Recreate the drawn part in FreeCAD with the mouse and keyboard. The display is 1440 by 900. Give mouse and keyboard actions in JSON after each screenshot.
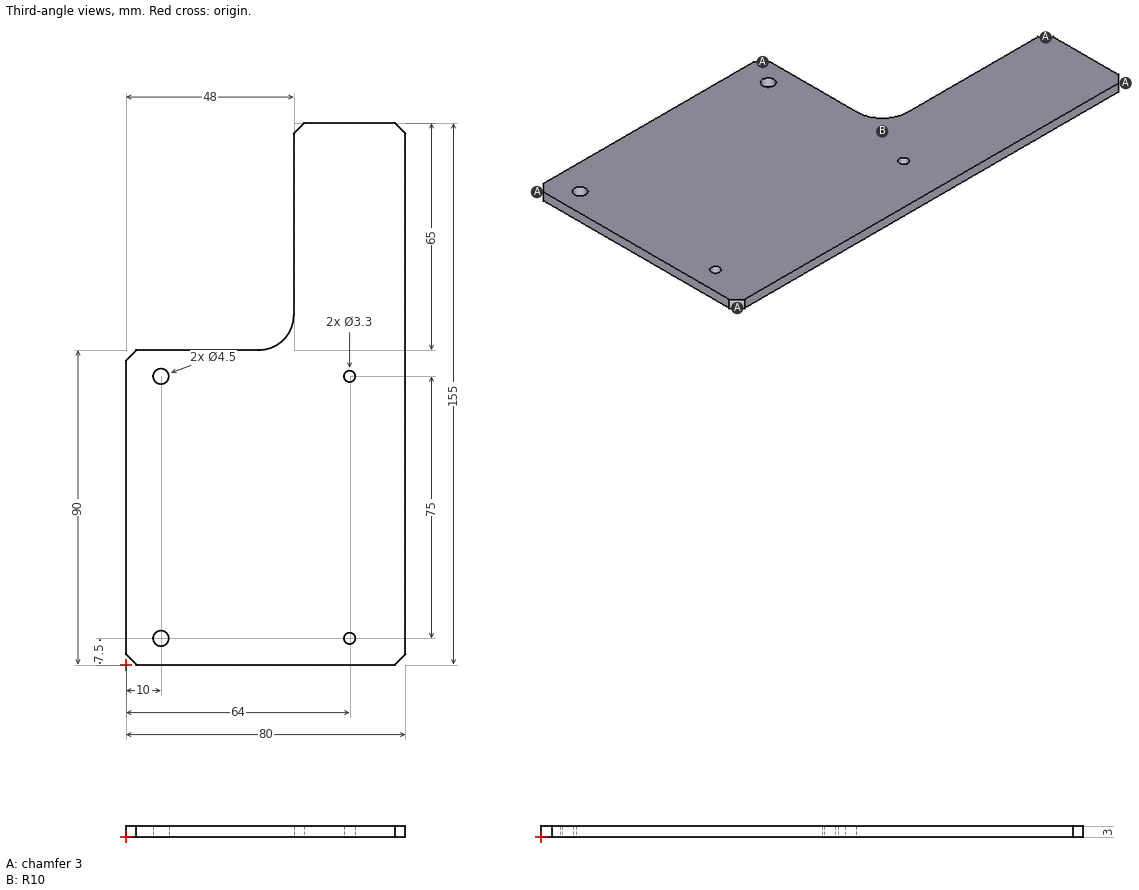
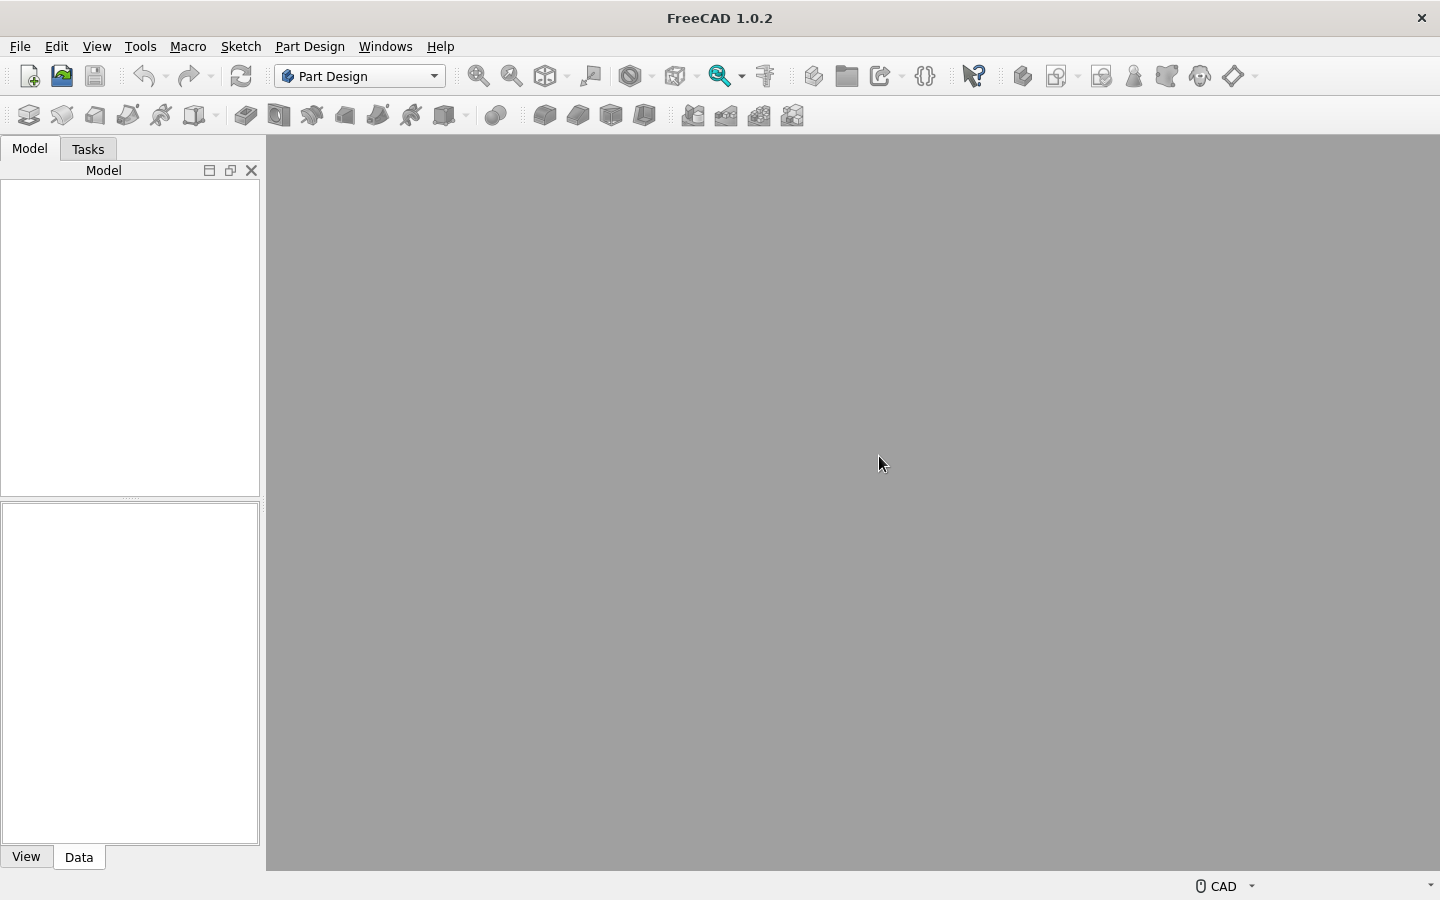
{"action": "left_click", "coordinate": [29, 76]}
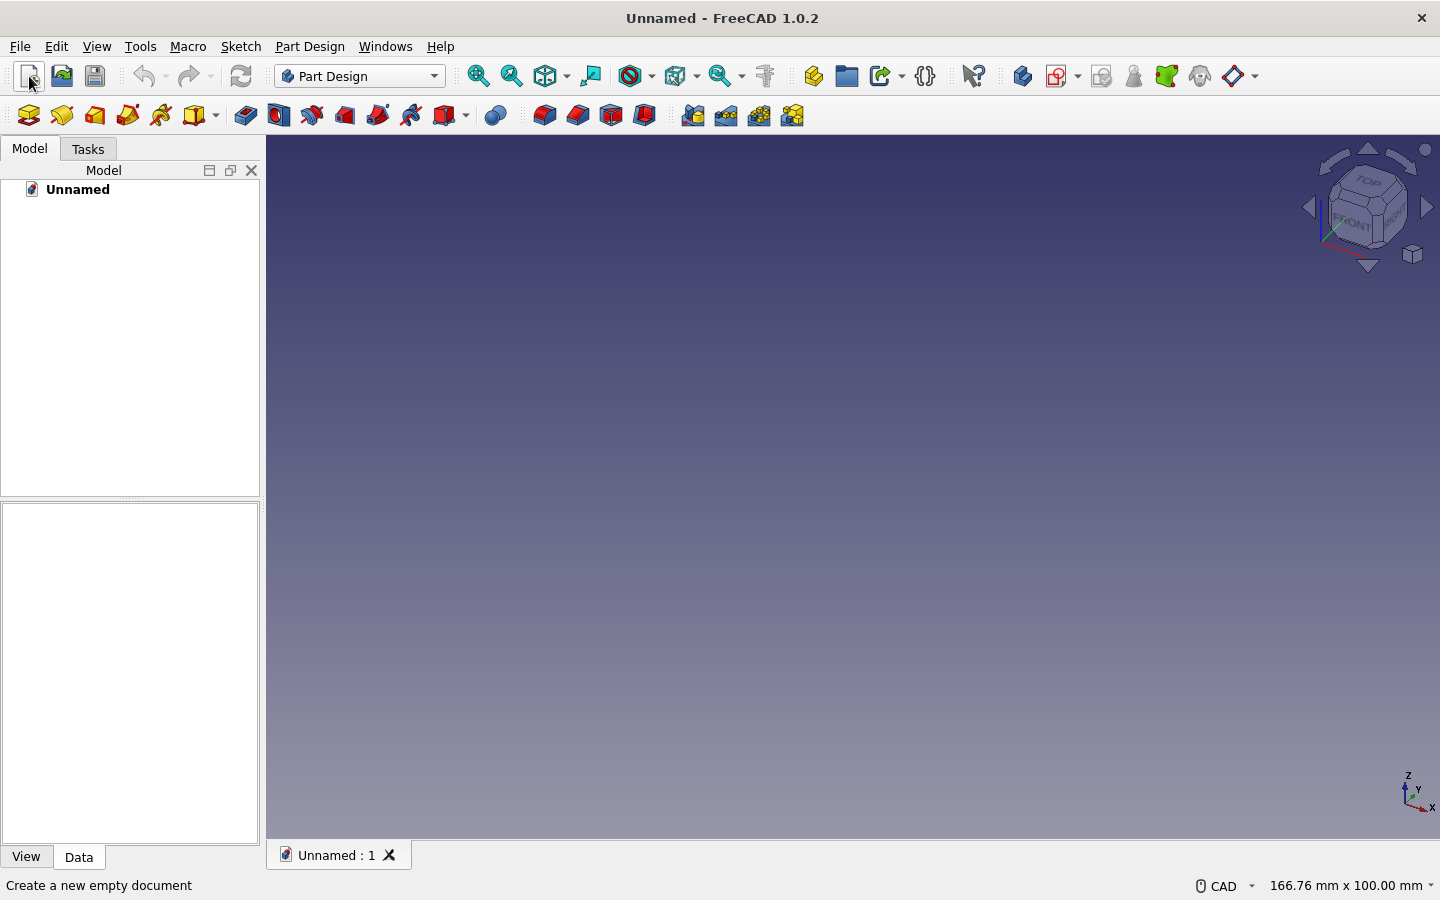
{"action": "left_click", "coordinate": [1056, 76]}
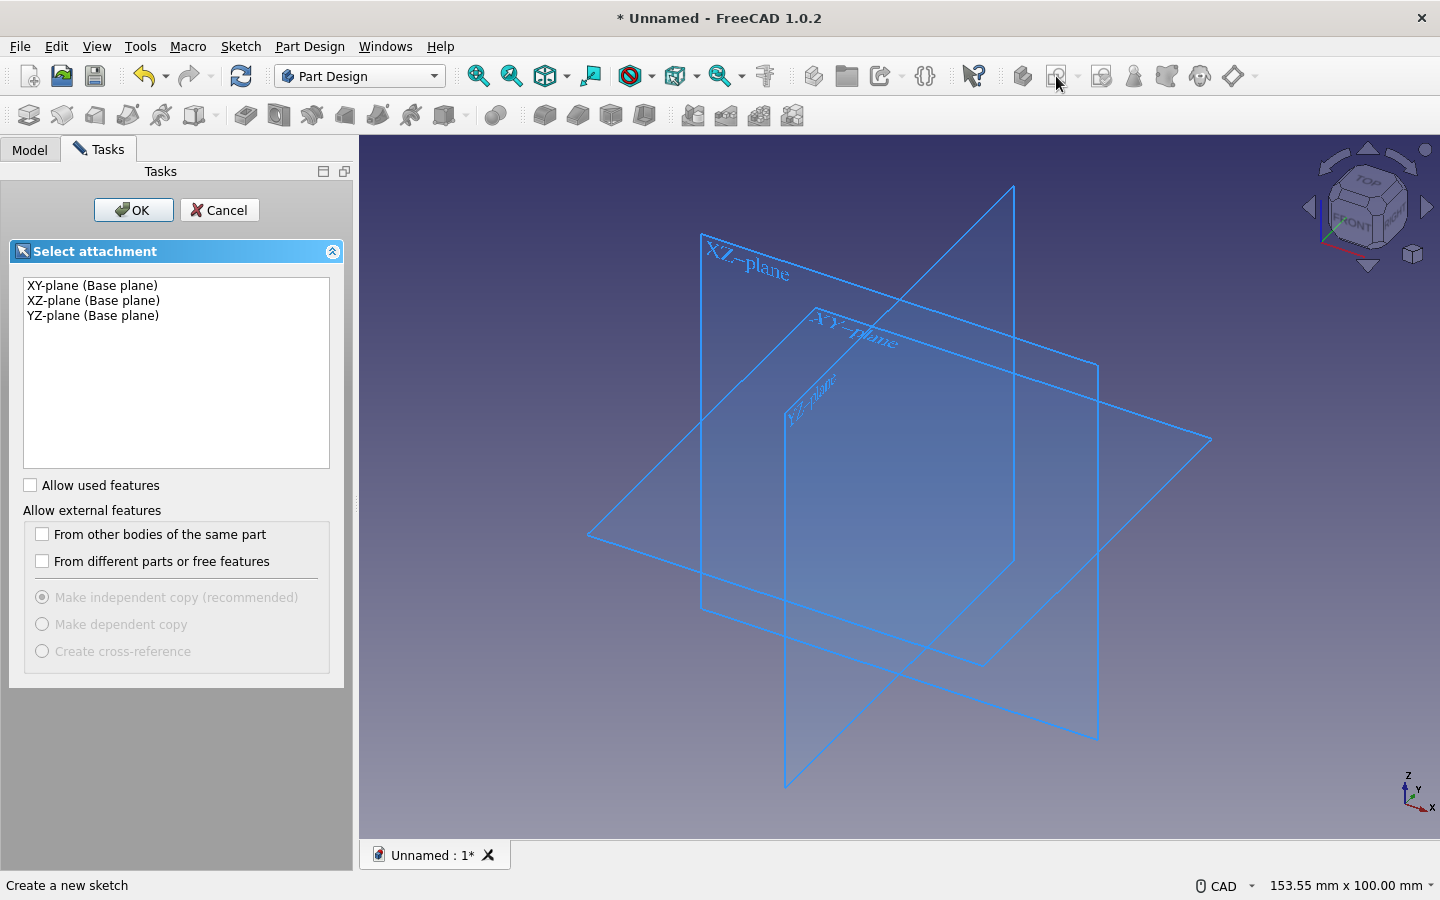
{"action": "left_click", "coordinate": [84, 286]}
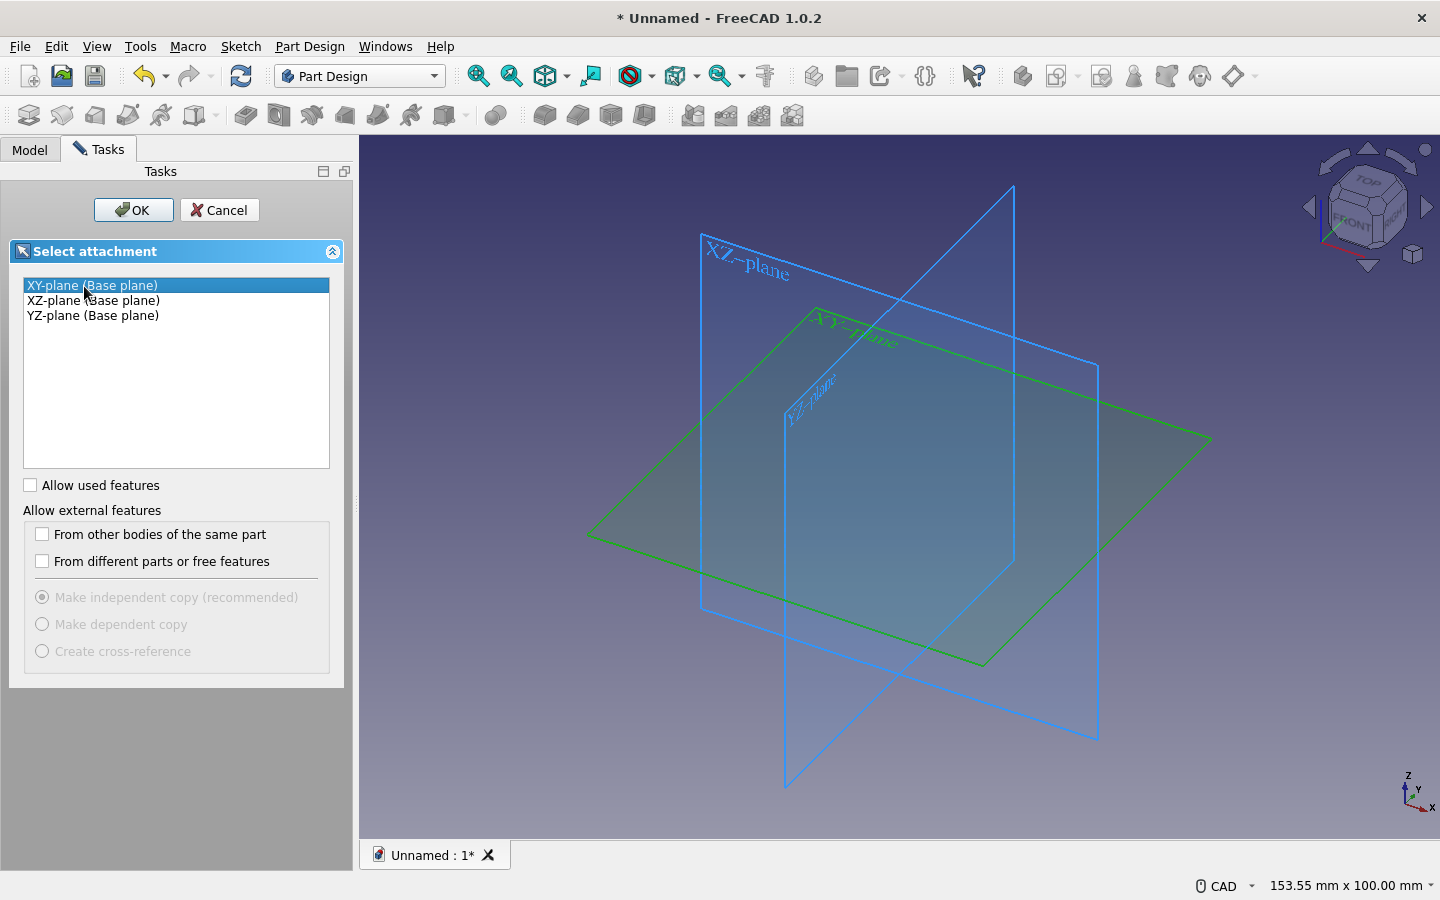
{"action": "left_click", "coordinate": [134, 210]}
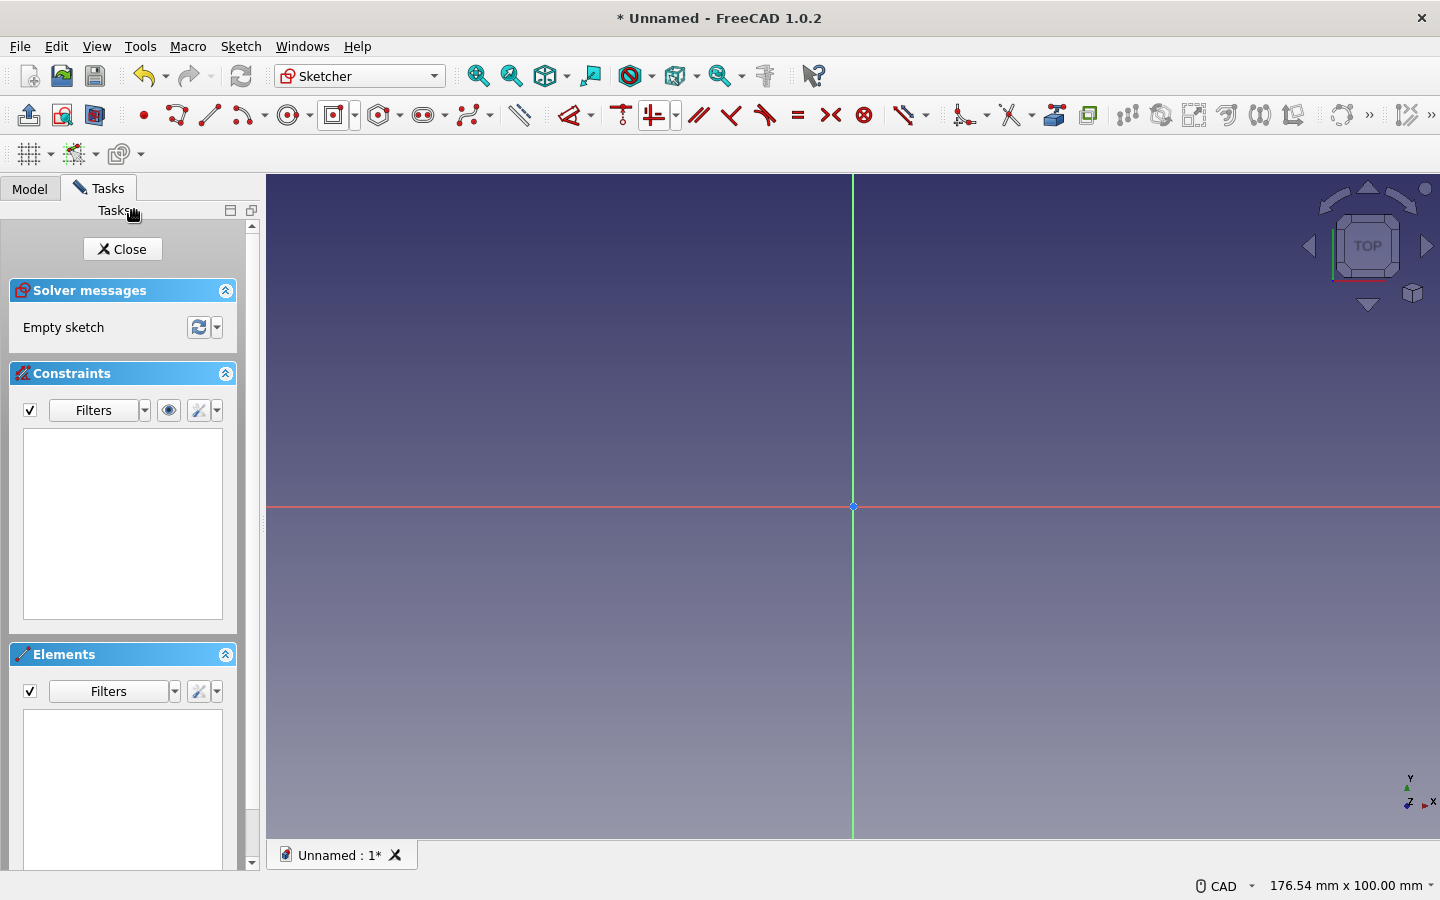
{"action": "scroll", "coordinate": [590, 806], "scroll_direction": "down", "scroll_amount": 5}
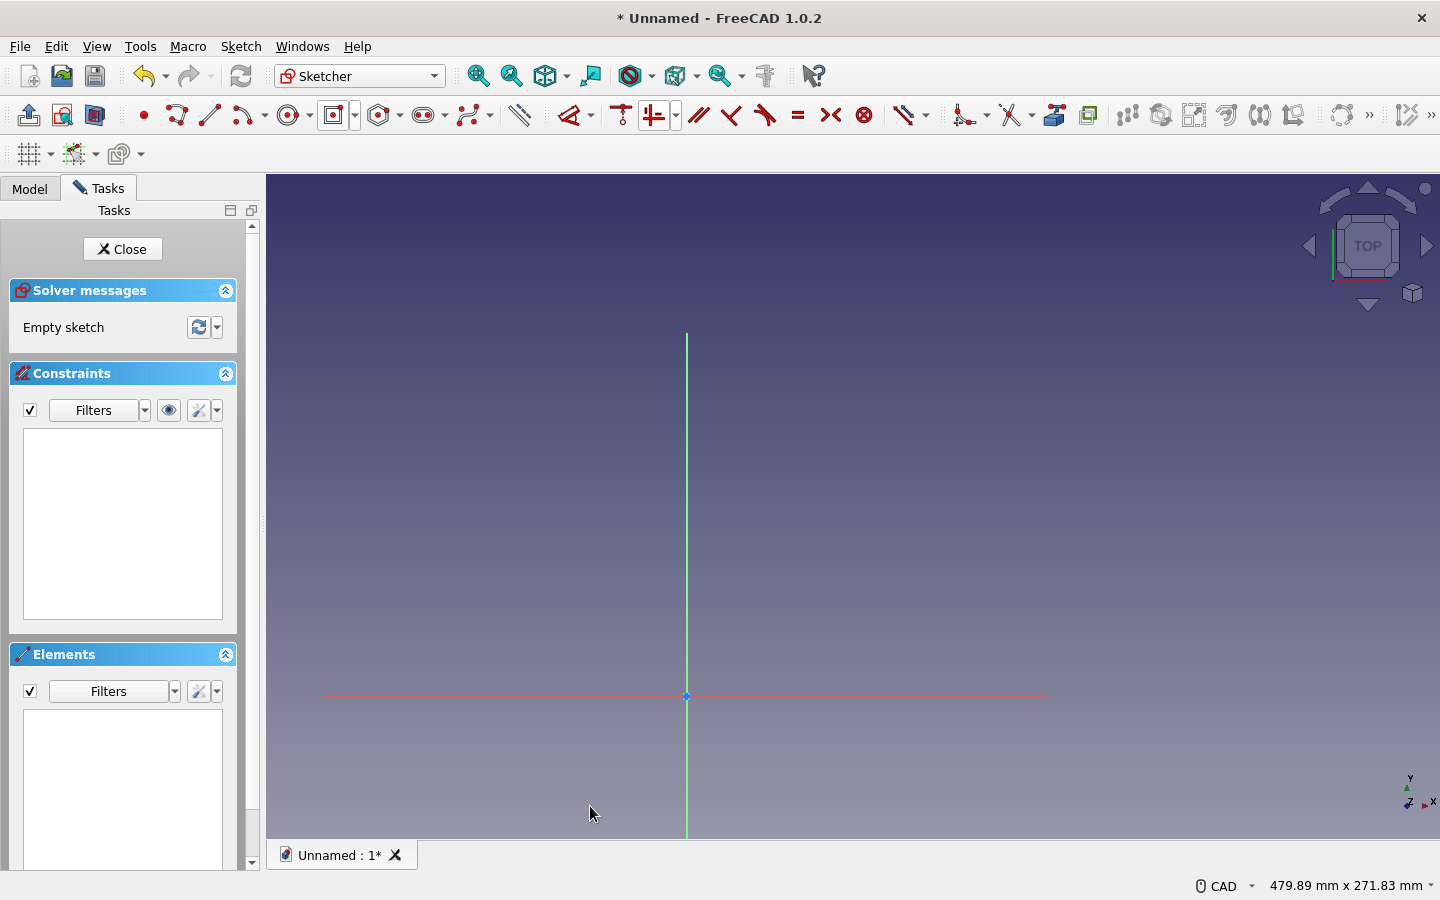
{"action": "left_click", "coordinate": [354, 116]}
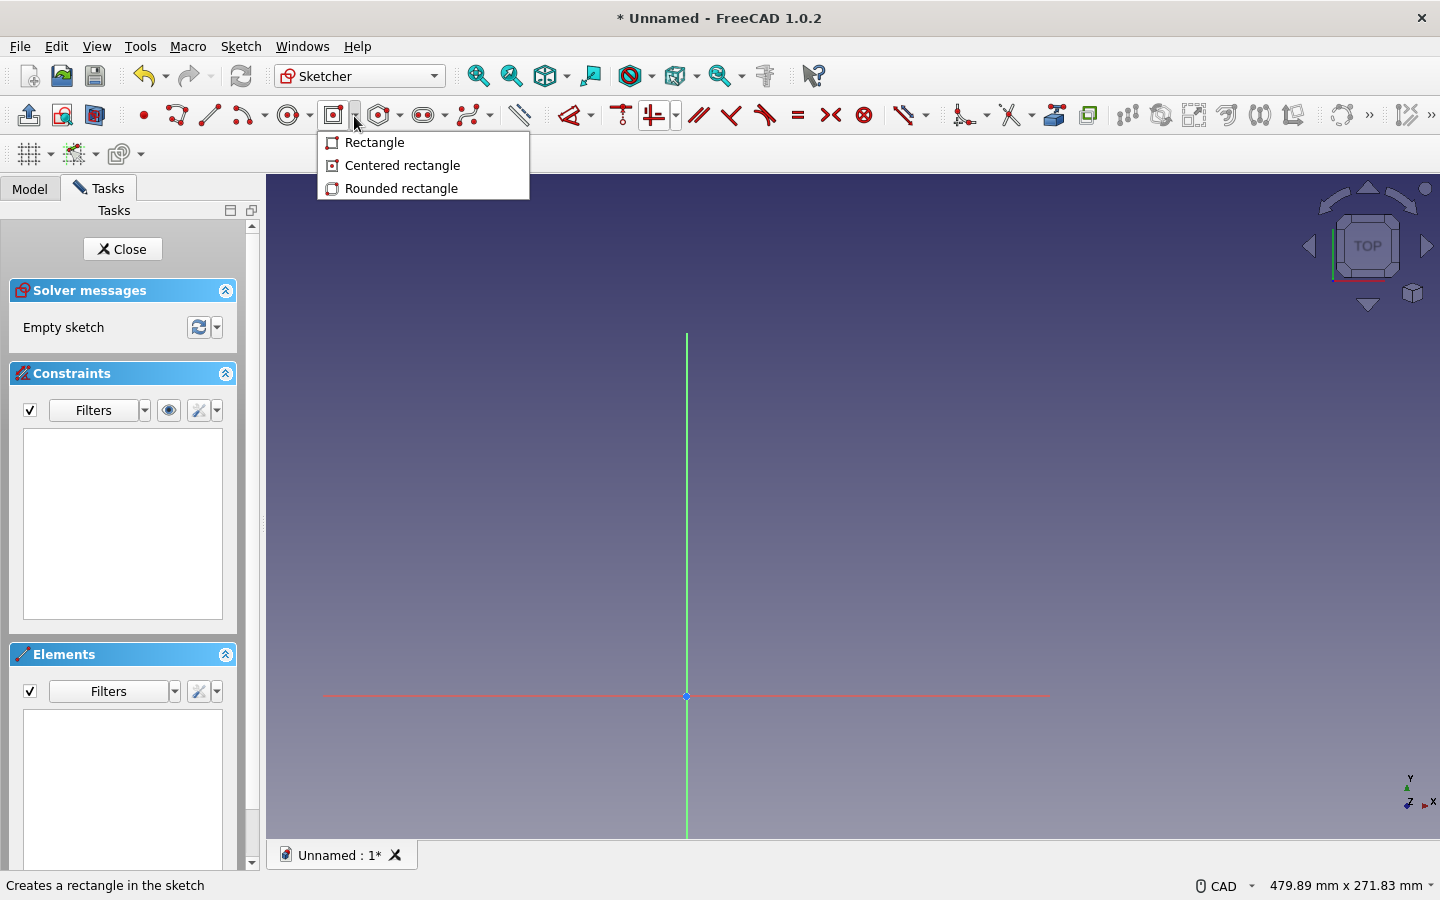
{"action": "left_click", "coordinate": [424, 142]}